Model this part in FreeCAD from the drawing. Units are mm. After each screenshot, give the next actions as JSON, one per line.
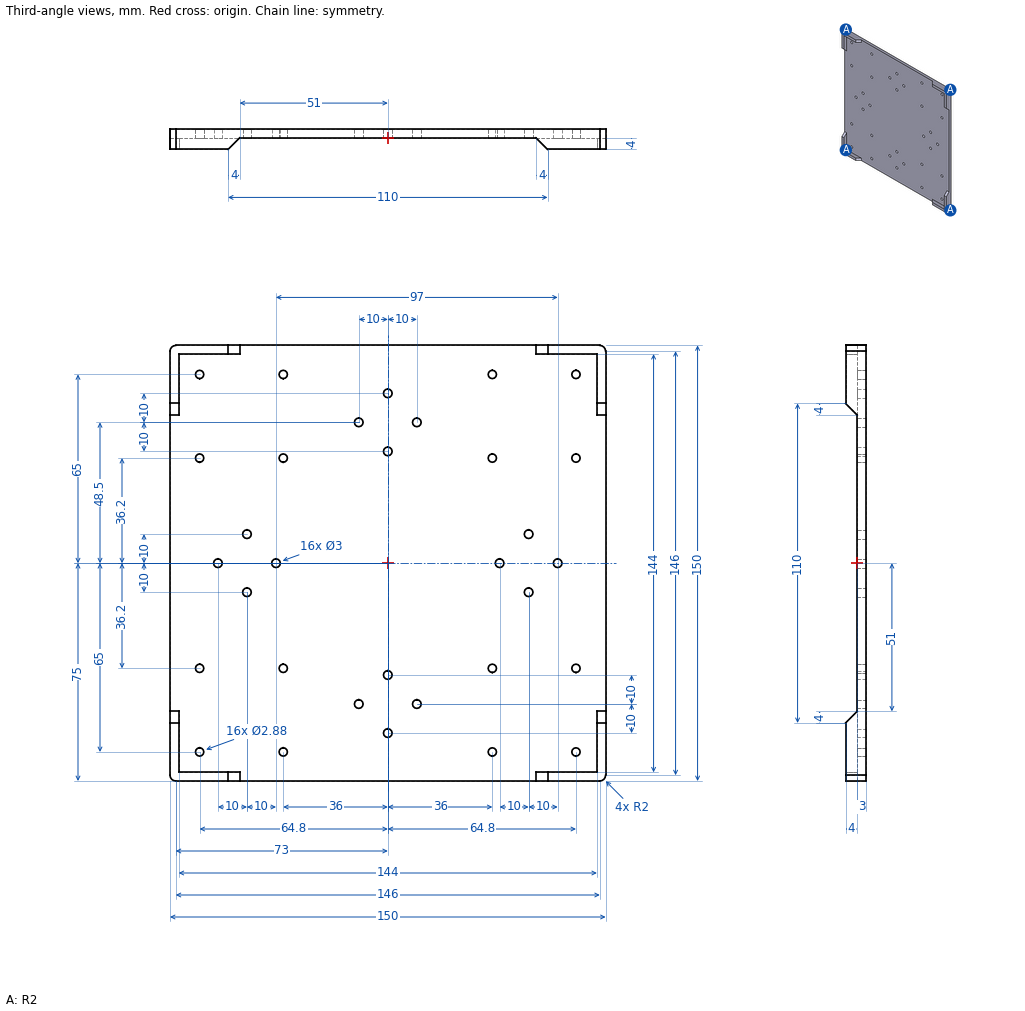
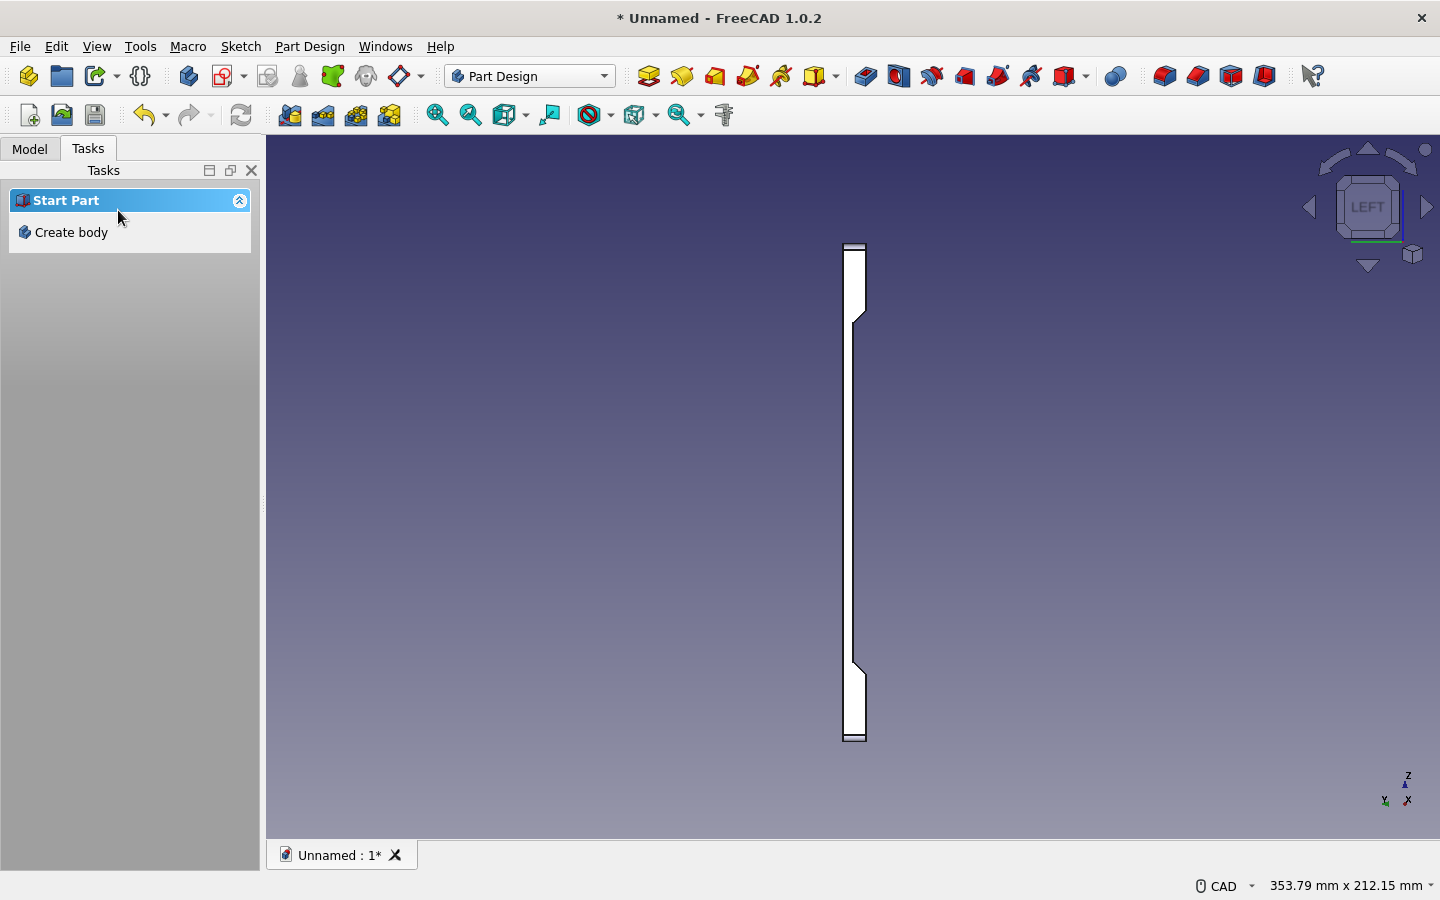
{"action": "key", "text": "0"}